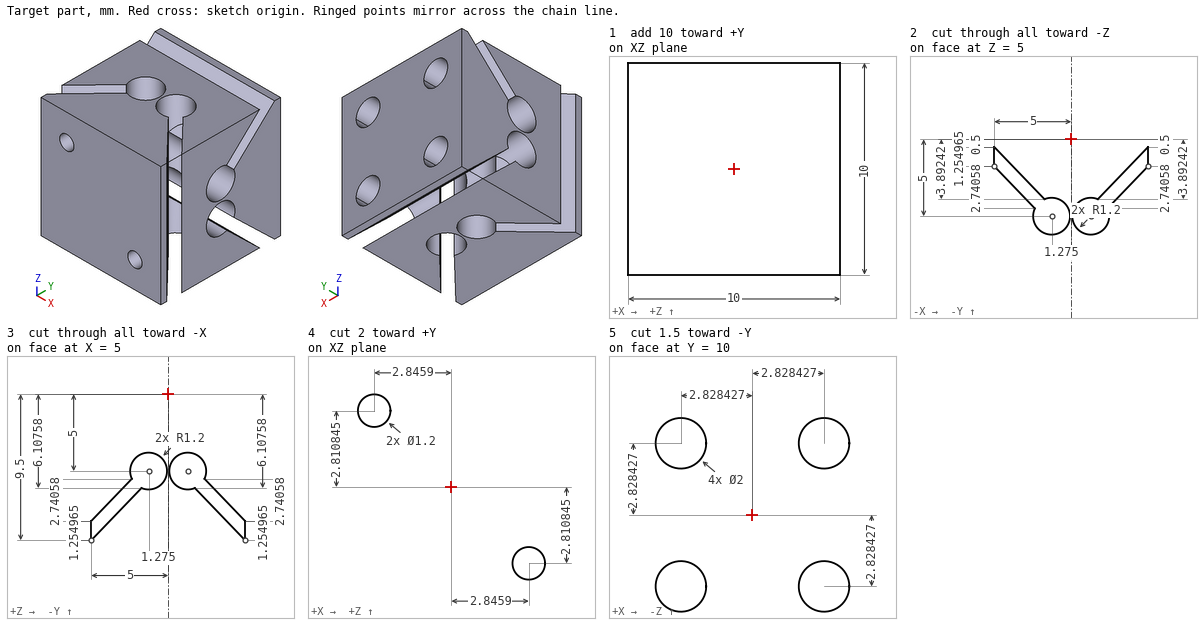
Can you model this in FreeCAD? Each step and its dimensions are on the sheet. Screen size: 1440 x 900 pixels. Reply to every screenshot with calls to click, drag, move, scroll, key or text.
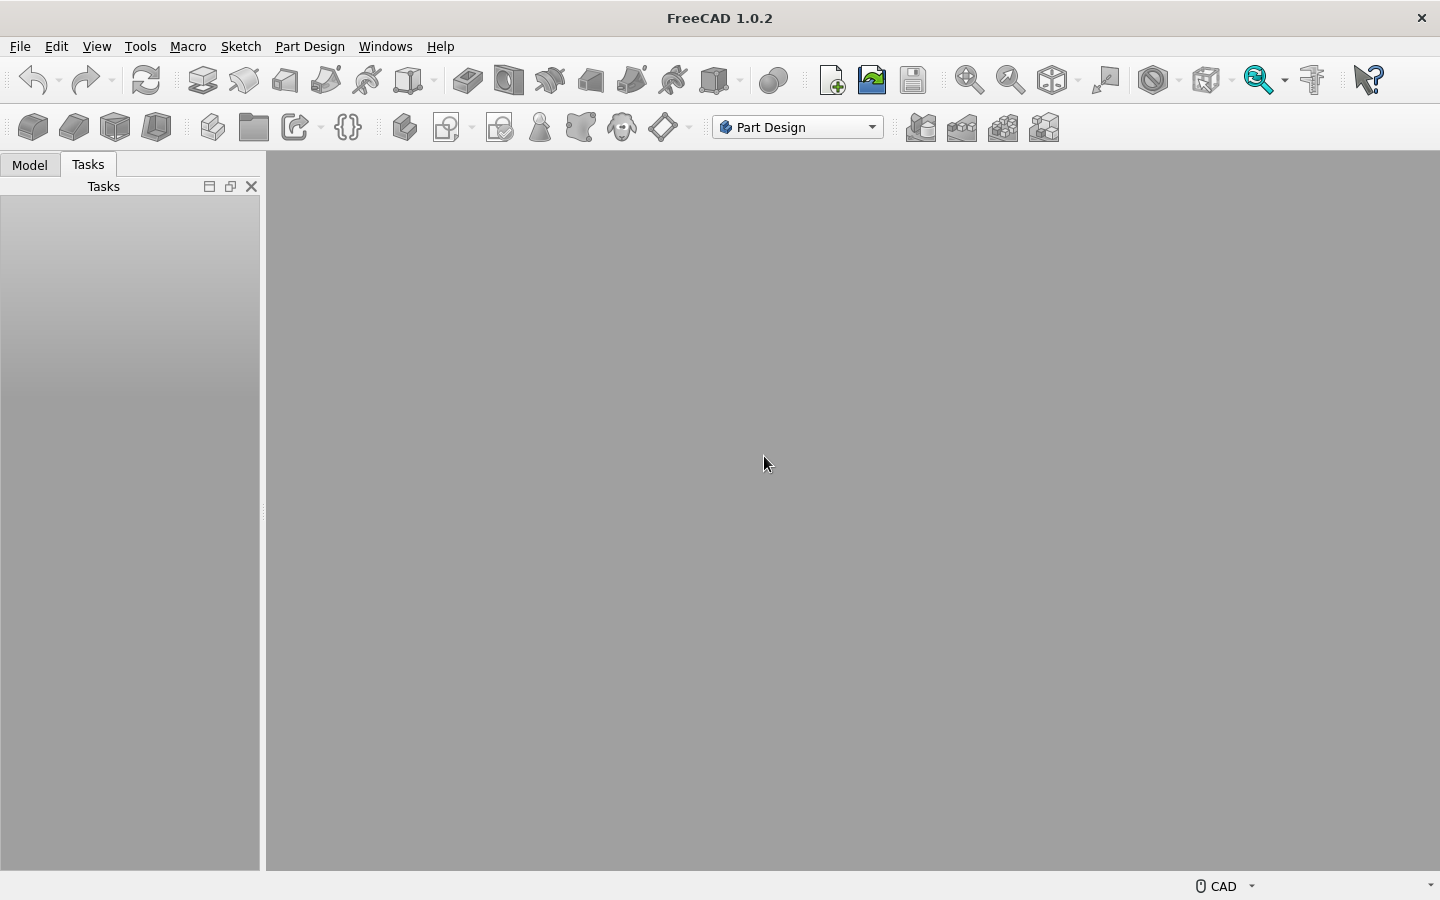
click(831, 80)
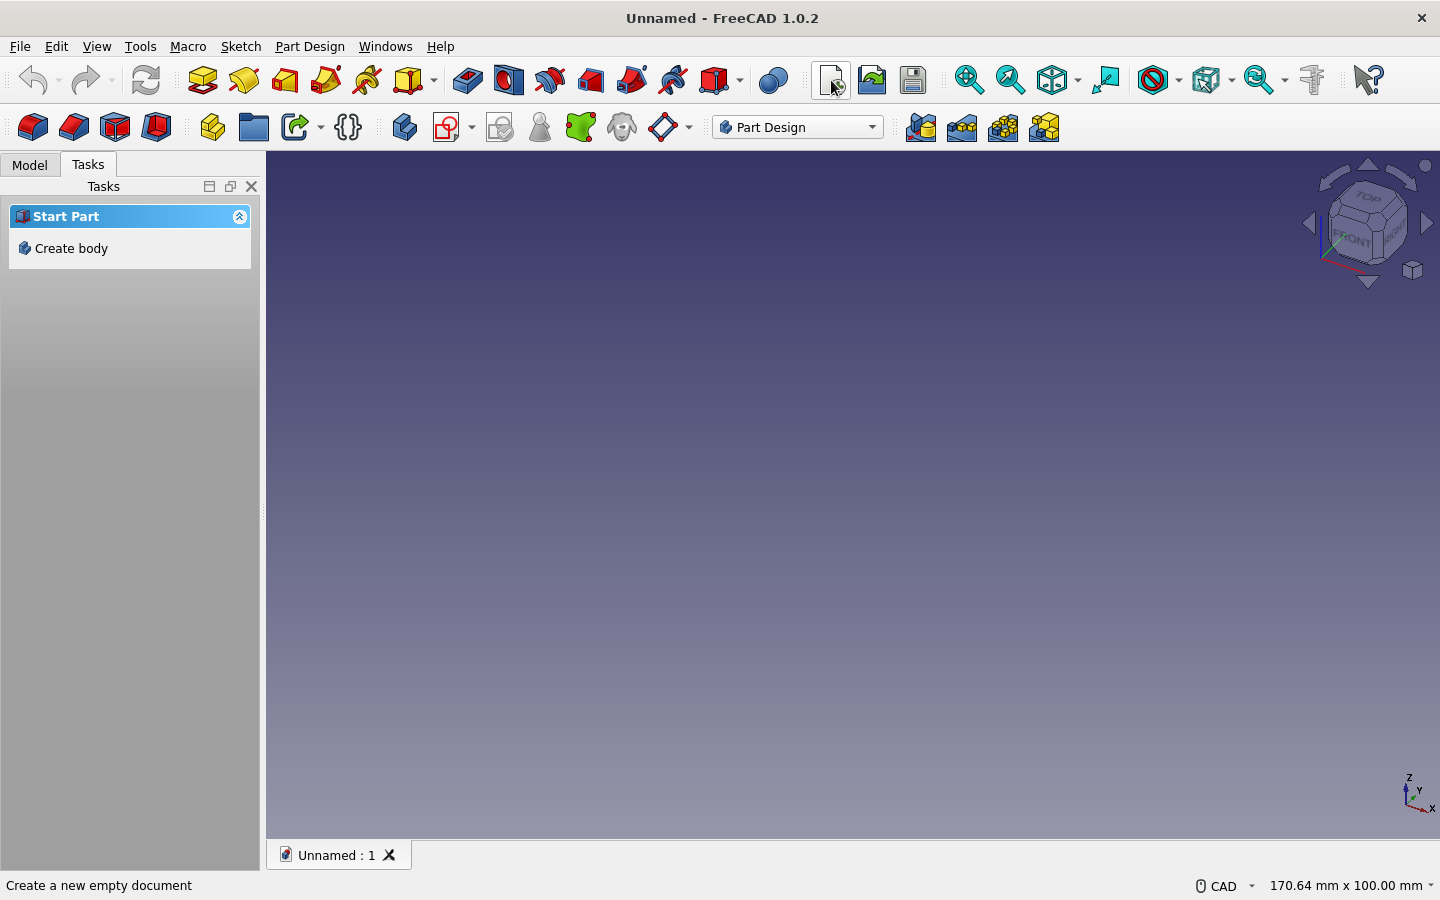
click(446, 128)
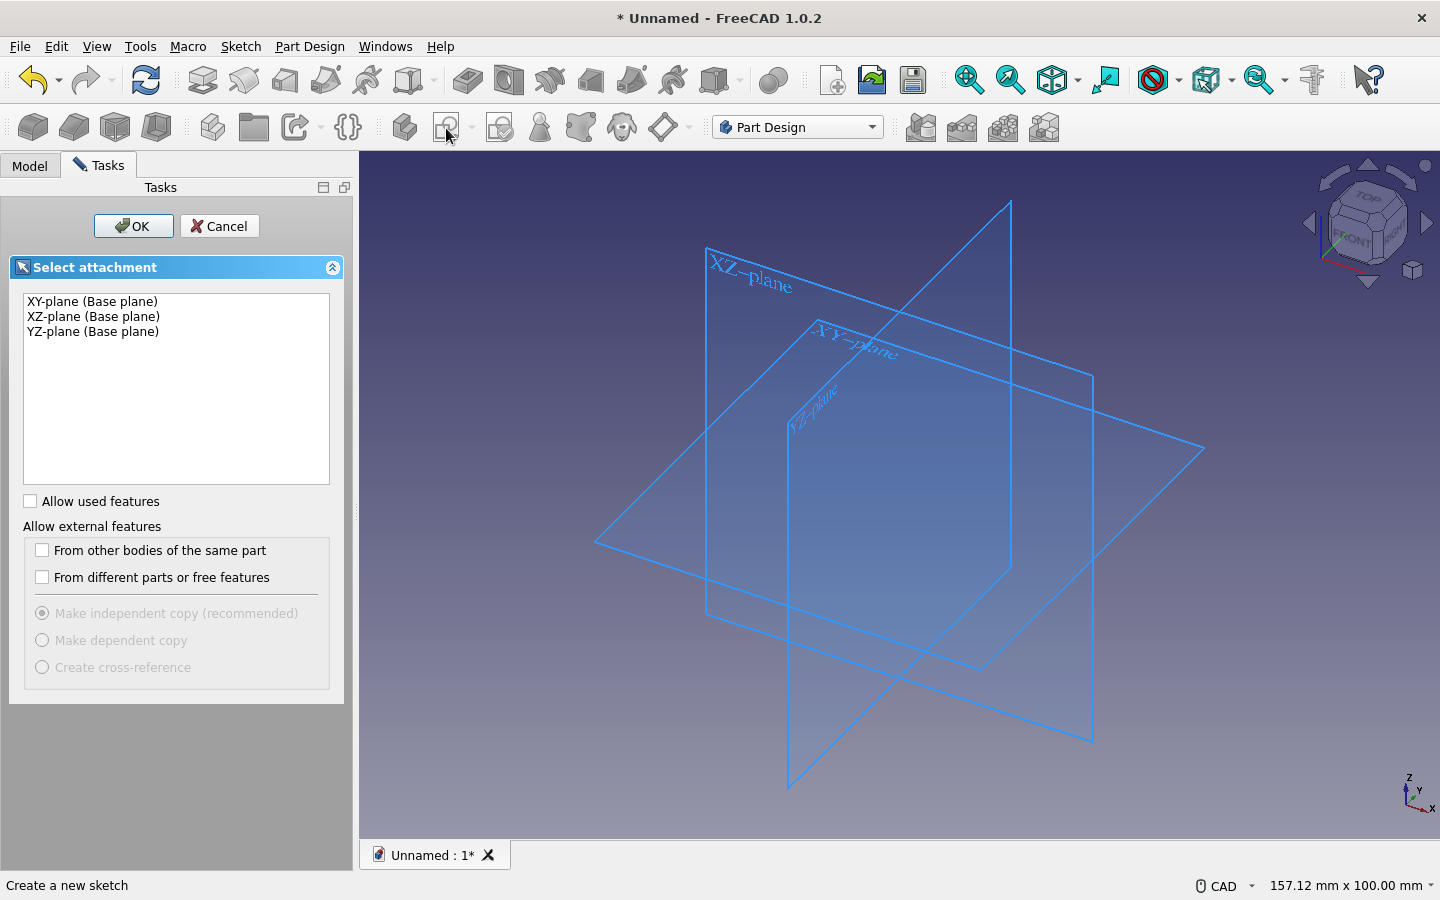
click(84, 316)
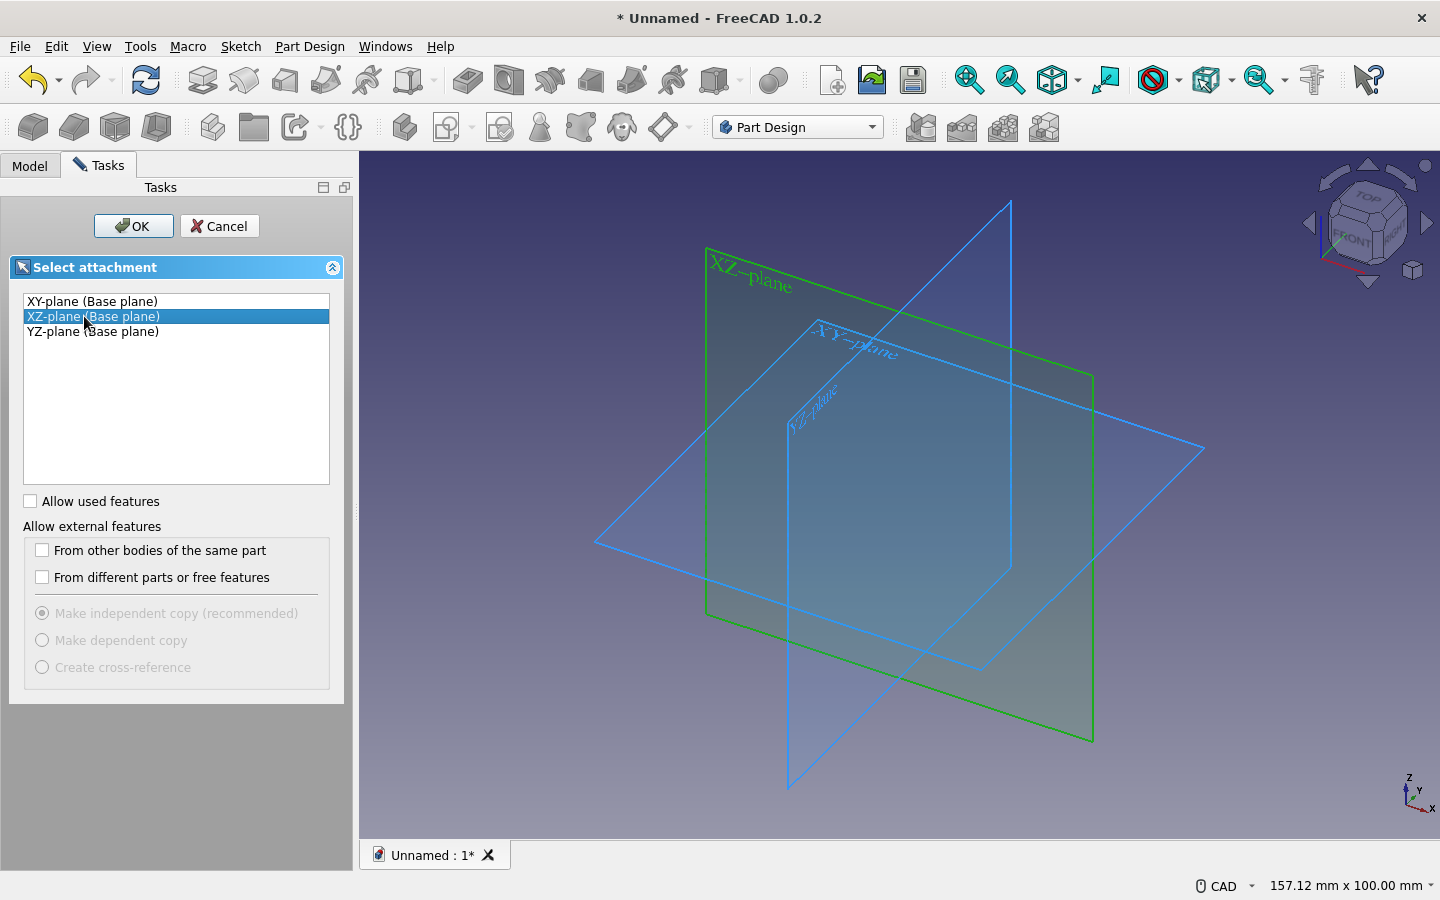
click(134, 226)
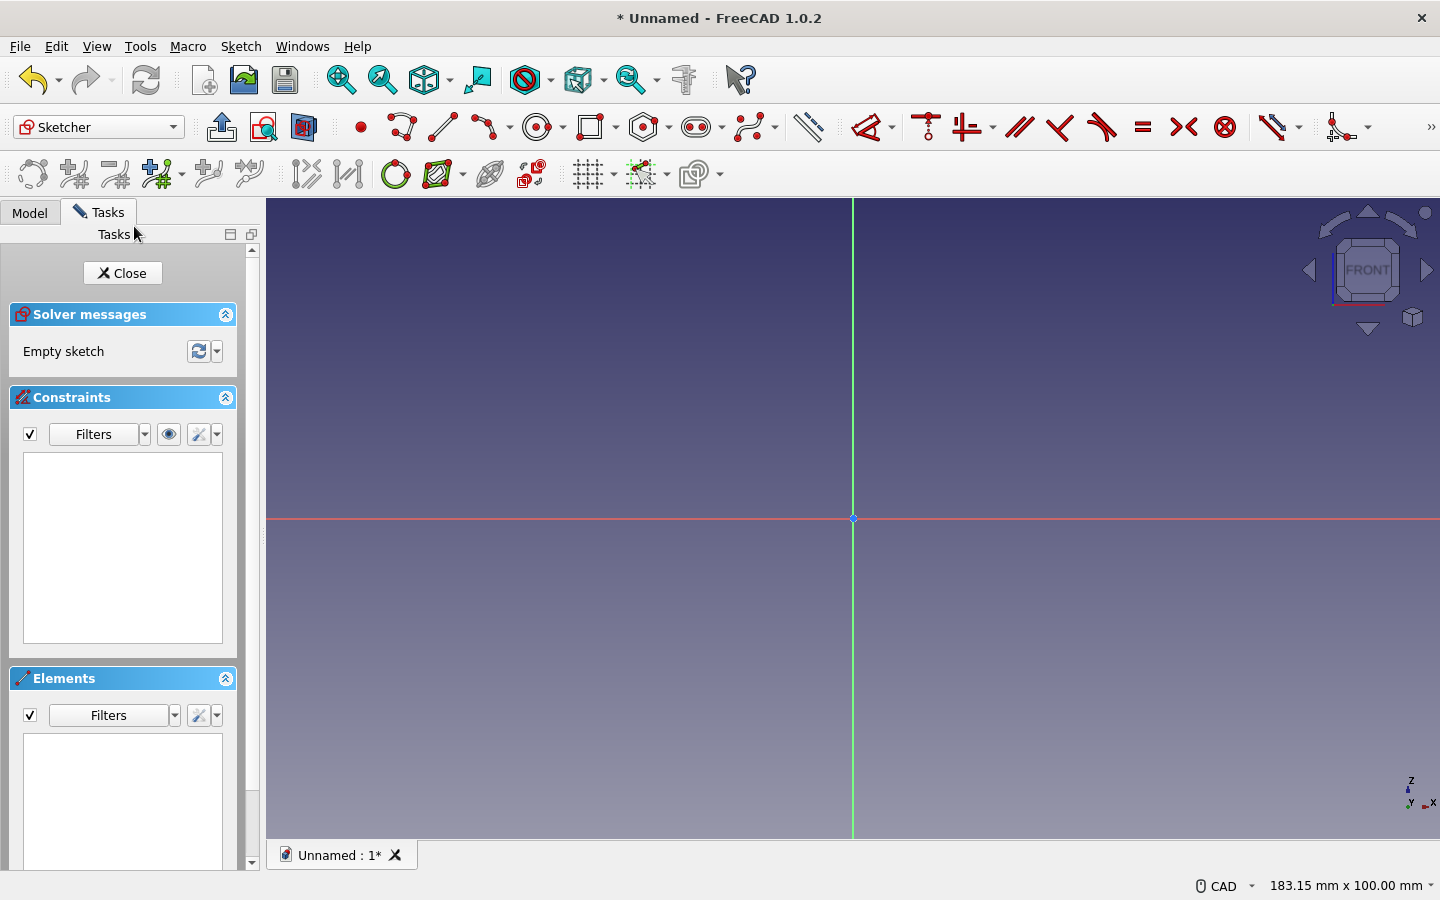
scroll(867, 518, up, 9)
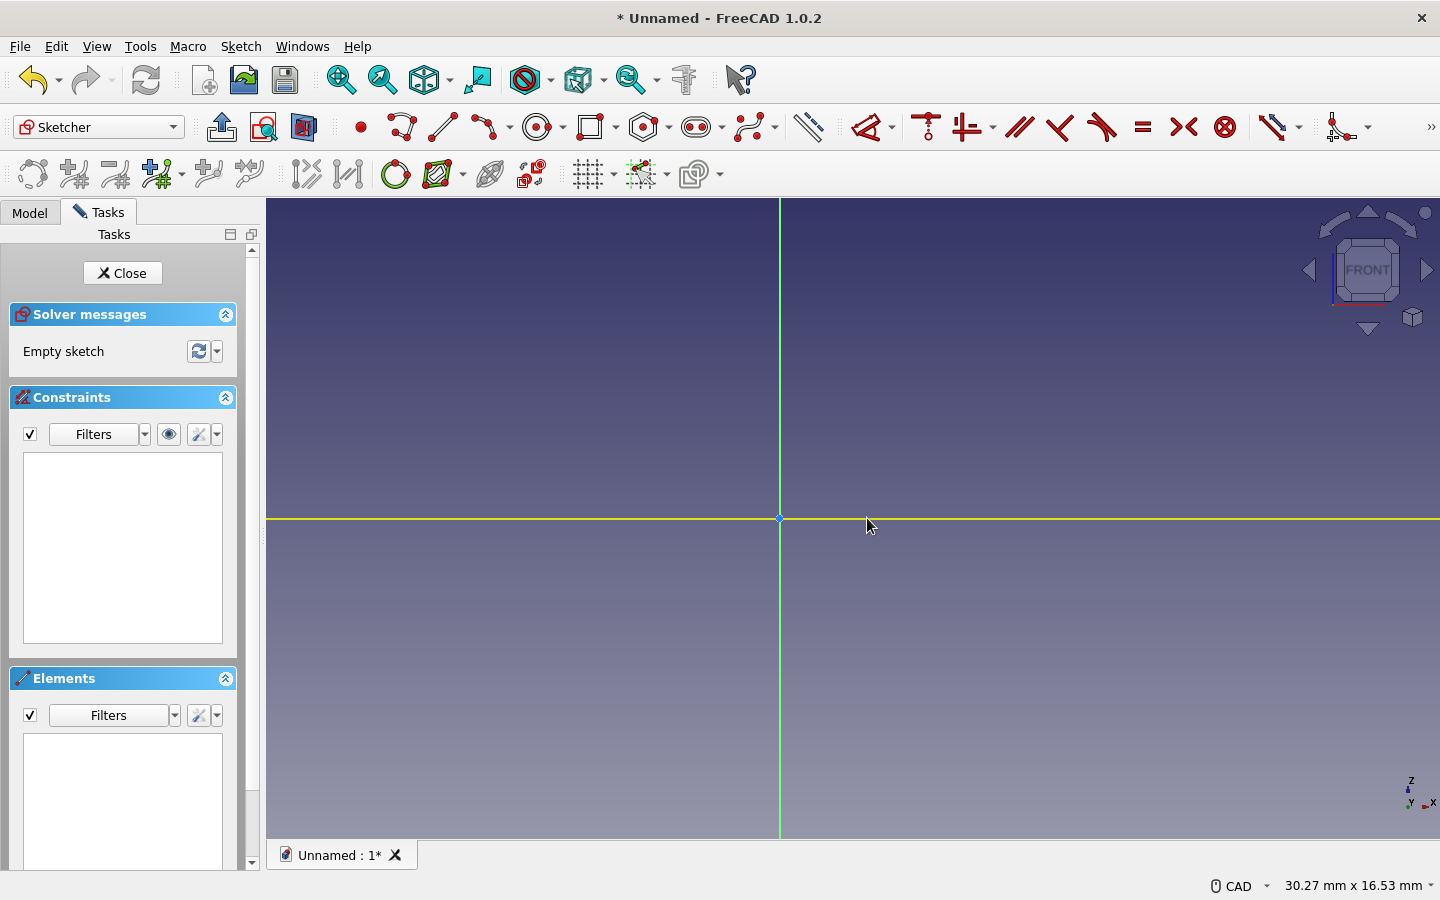
click(616, 128)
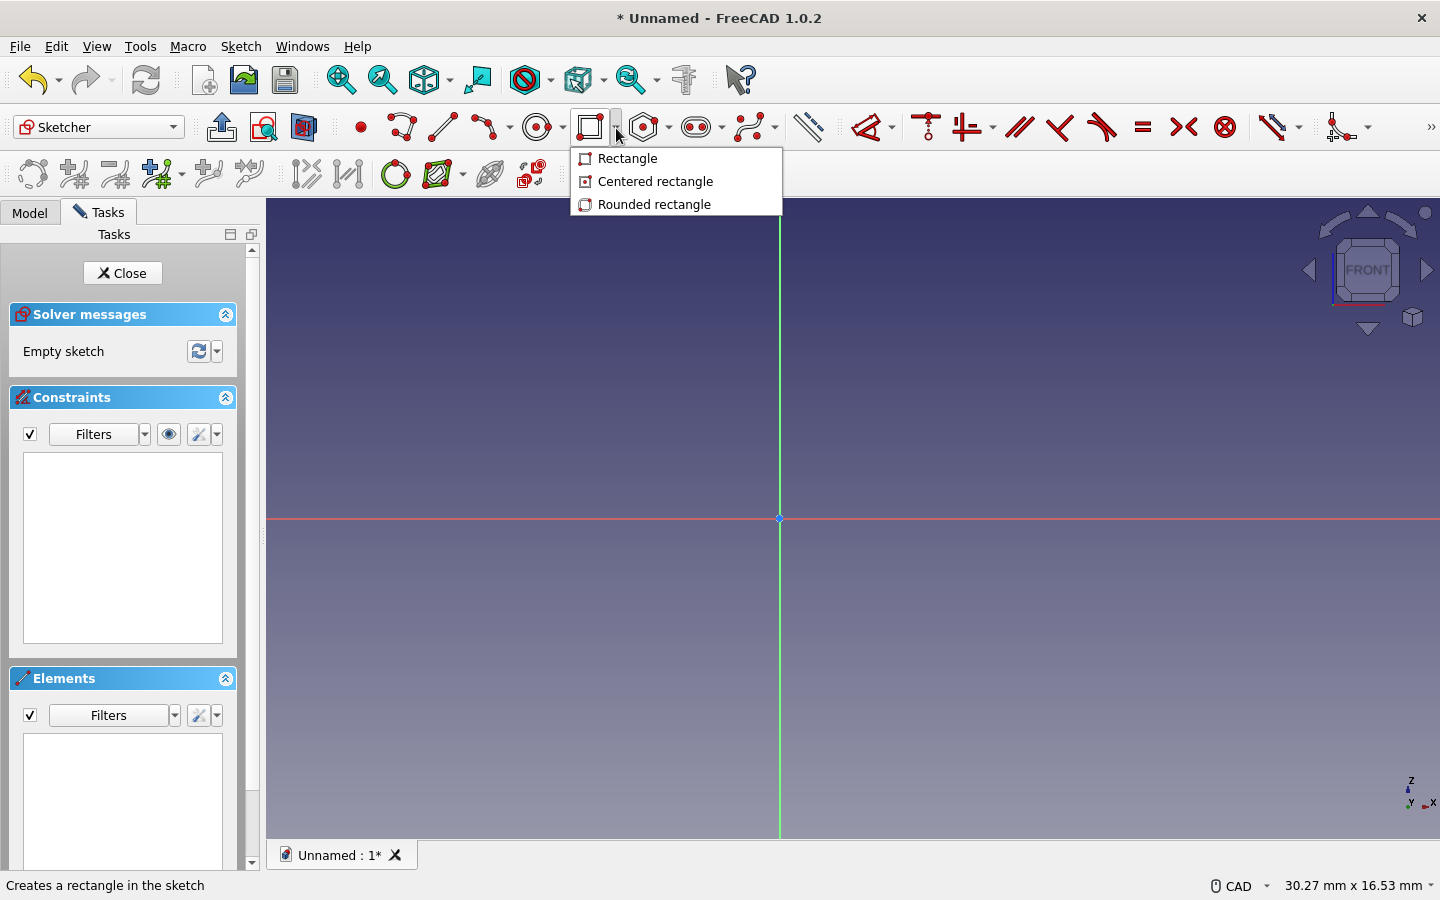
click(676, 182)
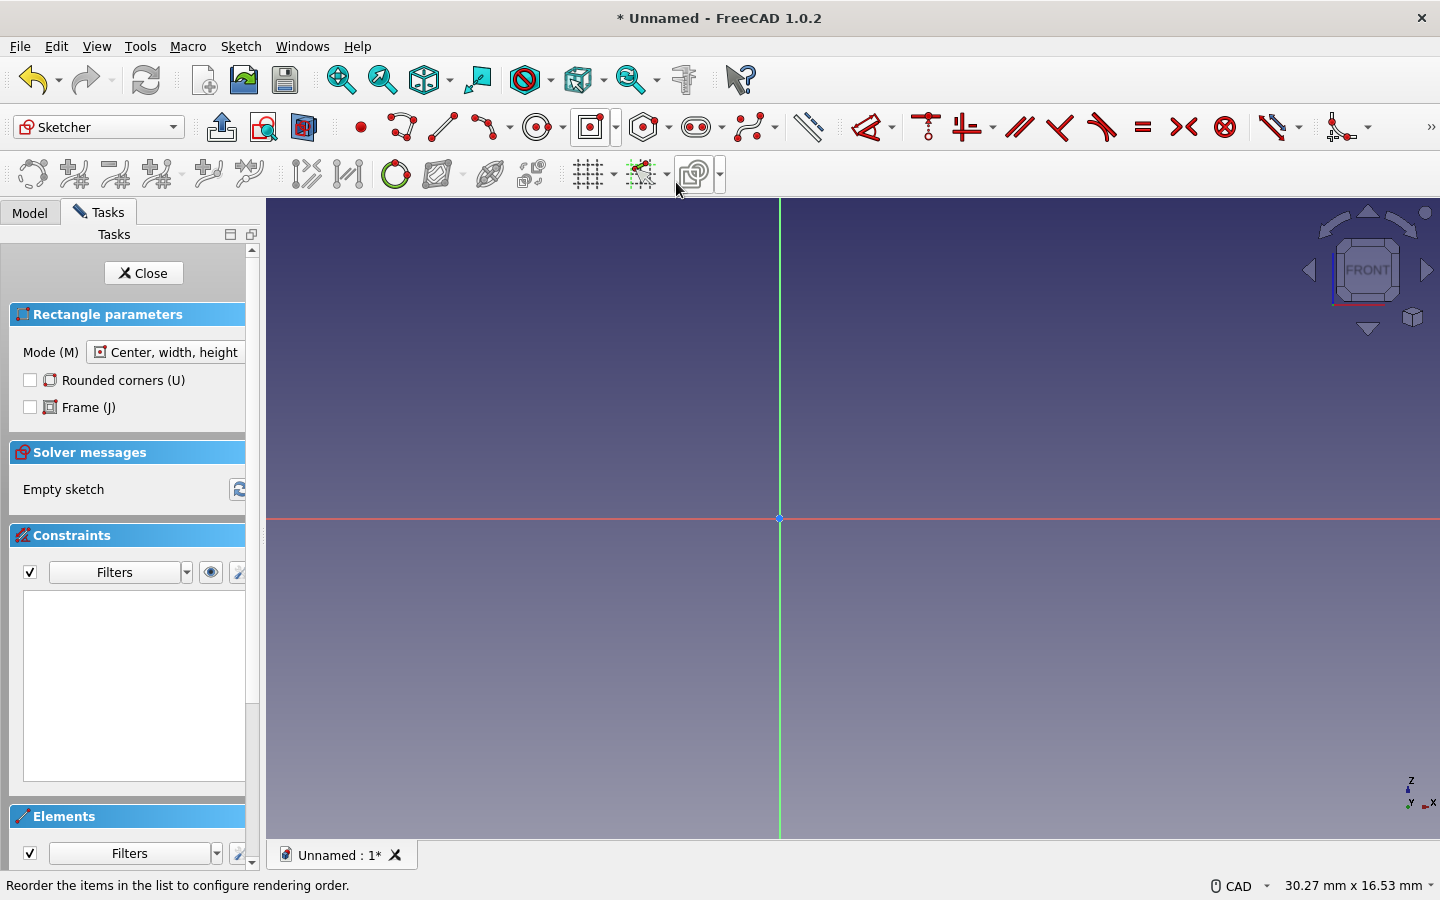
click(780, 518)
move(974, 325)